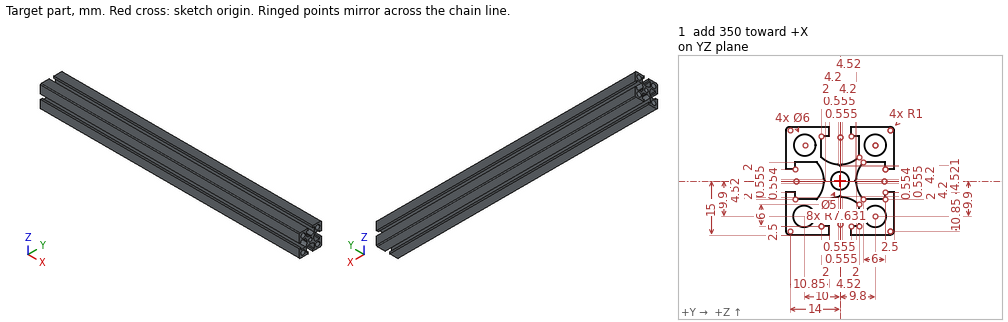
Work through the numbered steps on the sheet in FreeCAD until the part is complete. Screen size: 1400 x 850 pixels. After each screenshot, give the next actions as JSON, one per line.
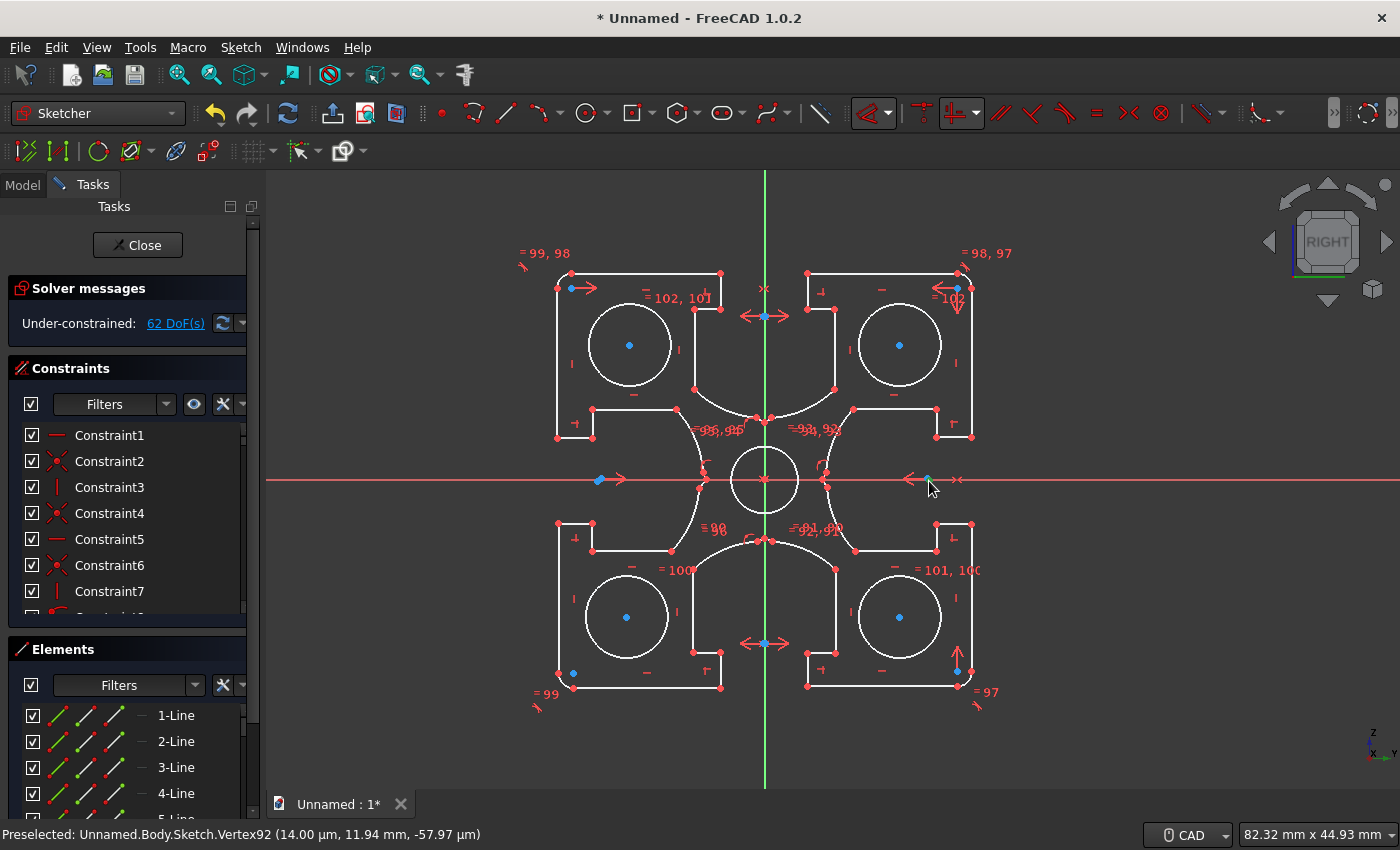
{"action": "scroll", "coordinate": [597, 481], "scroll_direction": "up", "scroll_amount": 6}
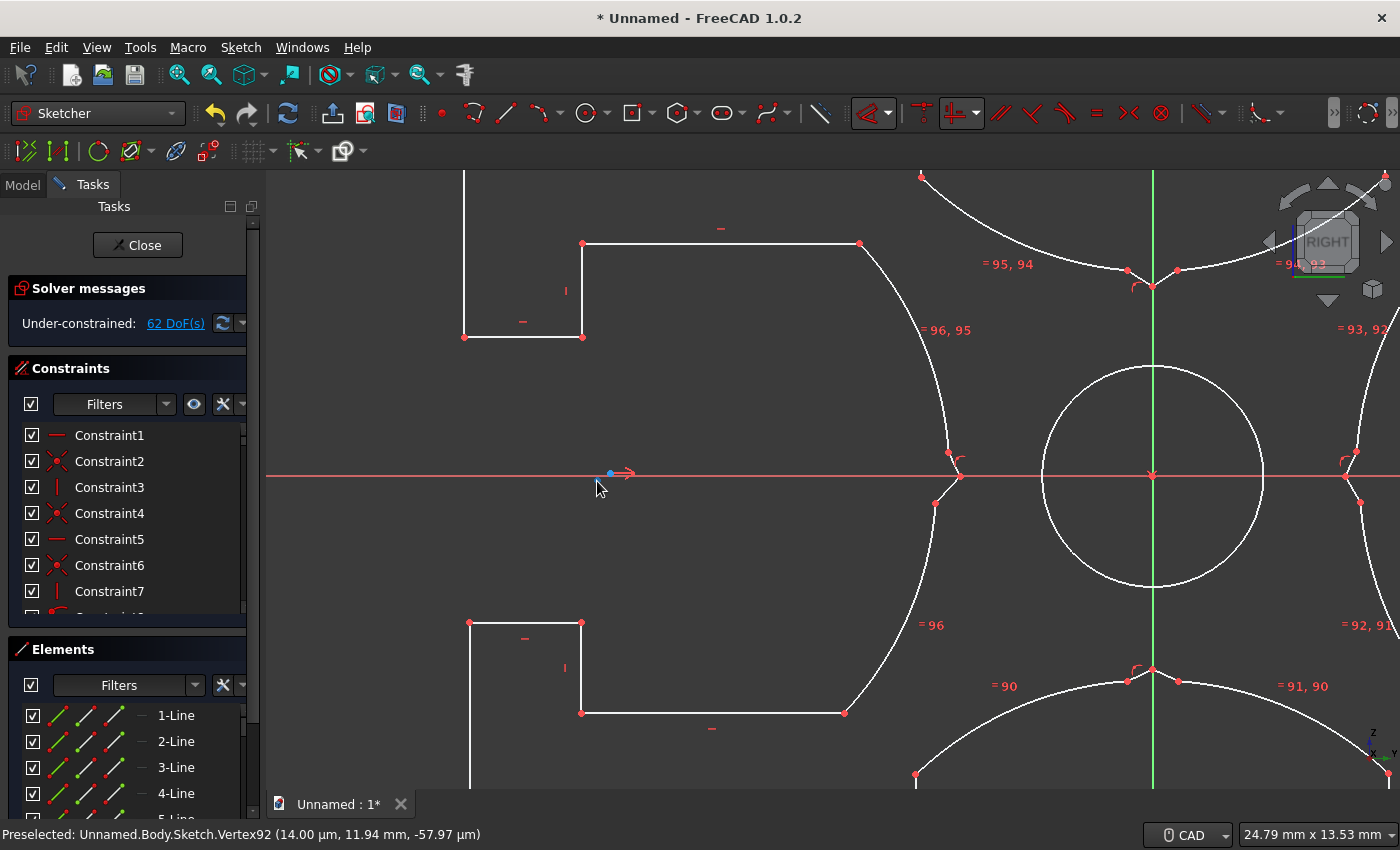
{"action": "left_click", "coordinate": [597, 481]}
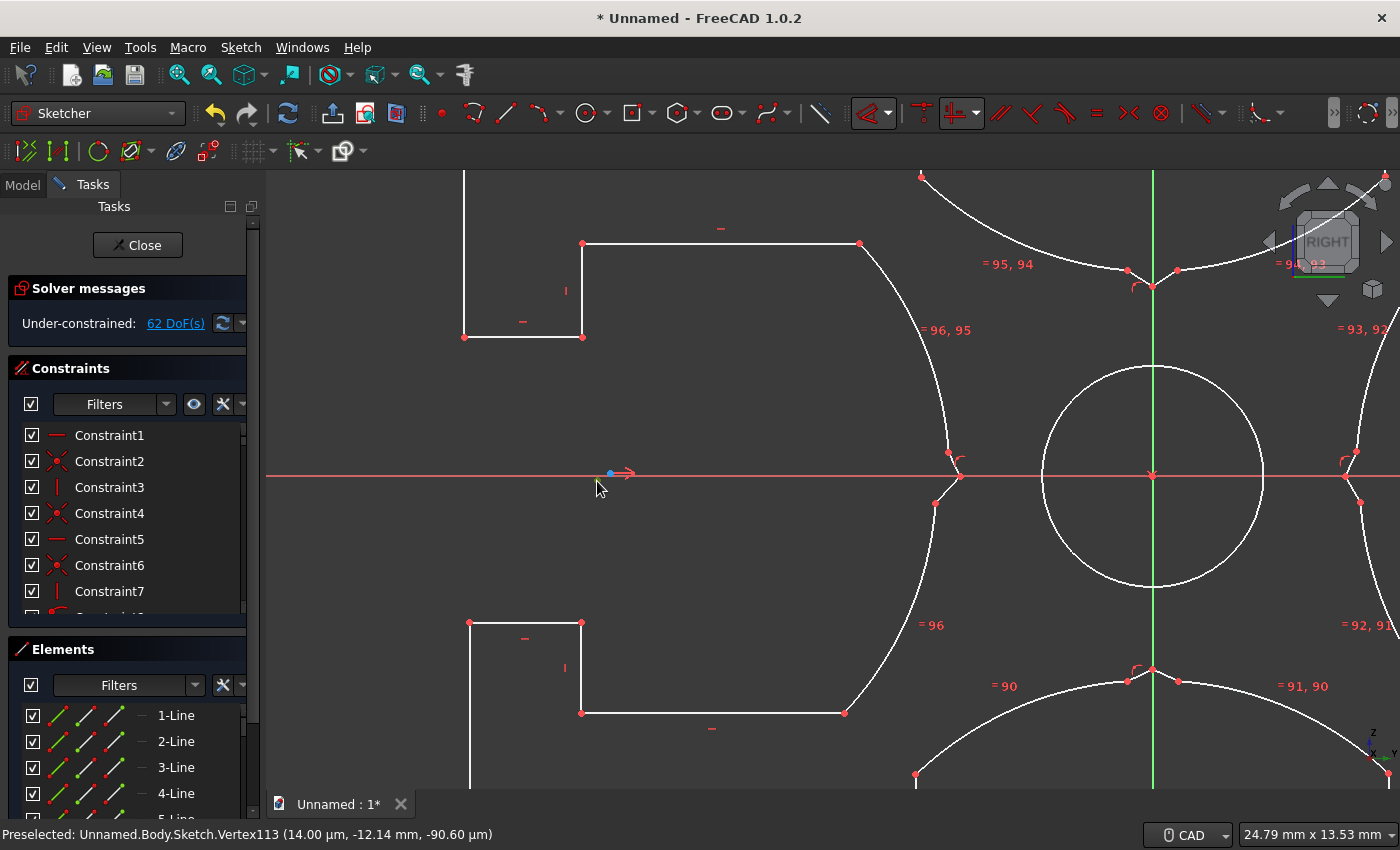
{"action": "left_click", "coordinate": [1153, 721]}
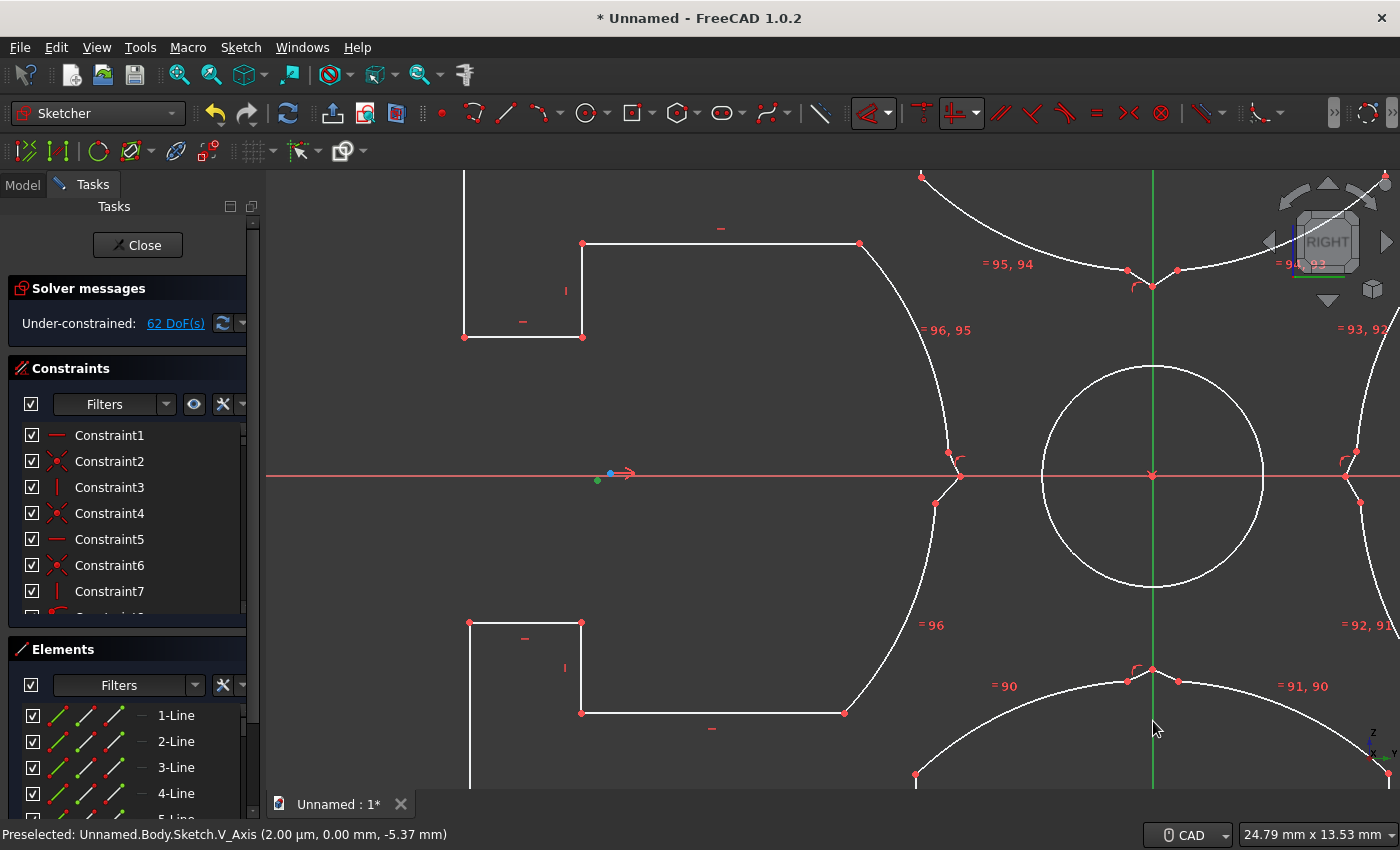
{"action": "left_click", "coordinate": [1130, 114]}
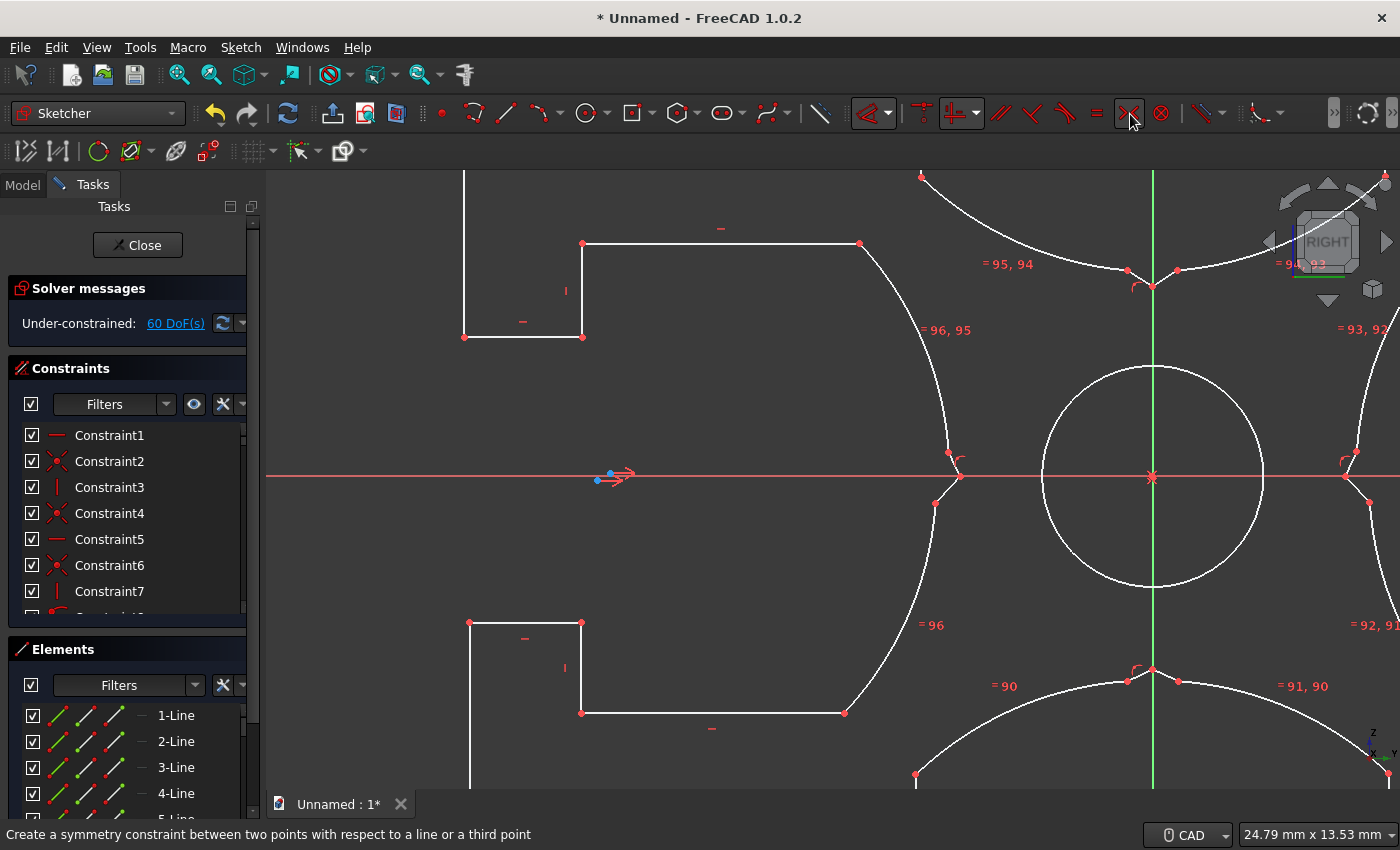
{"action": "scroll", "coordinate": [597, 481], "scroll_direction": "down", "scroll_amount": 6}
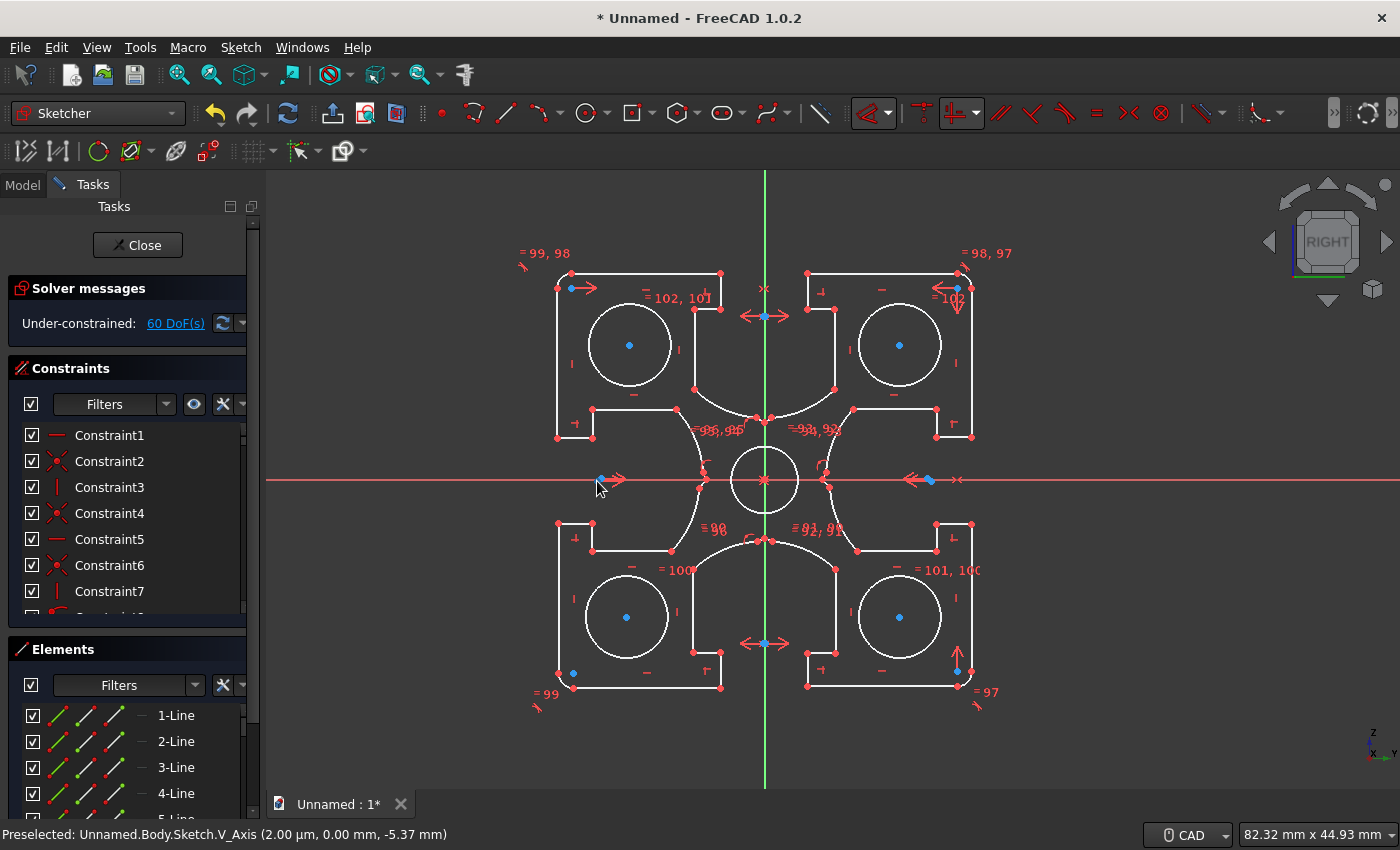
{"action": "left_click", "coordinate": [957, 672]}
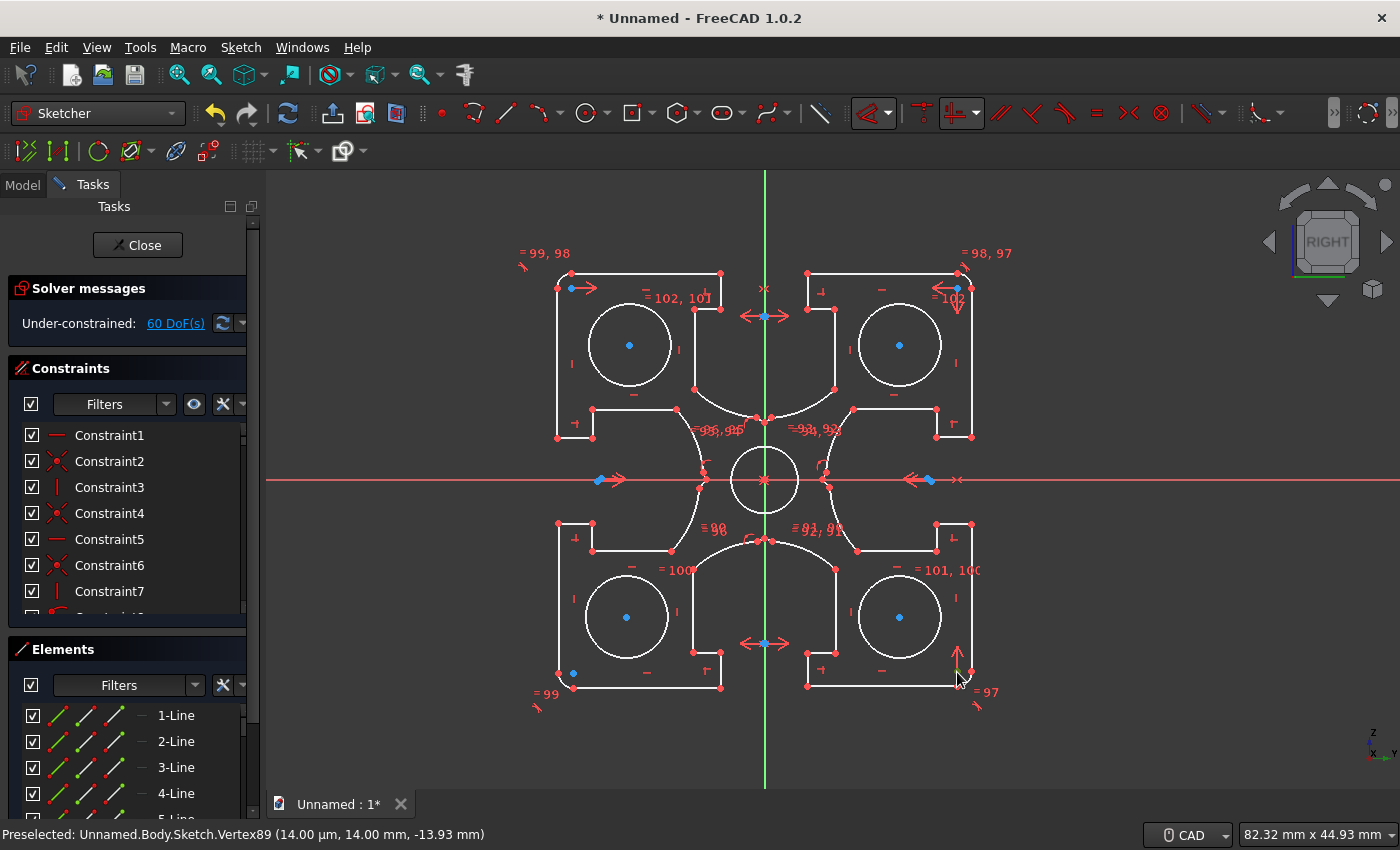
{"action": "left_click", "coordinate": [573, 674]}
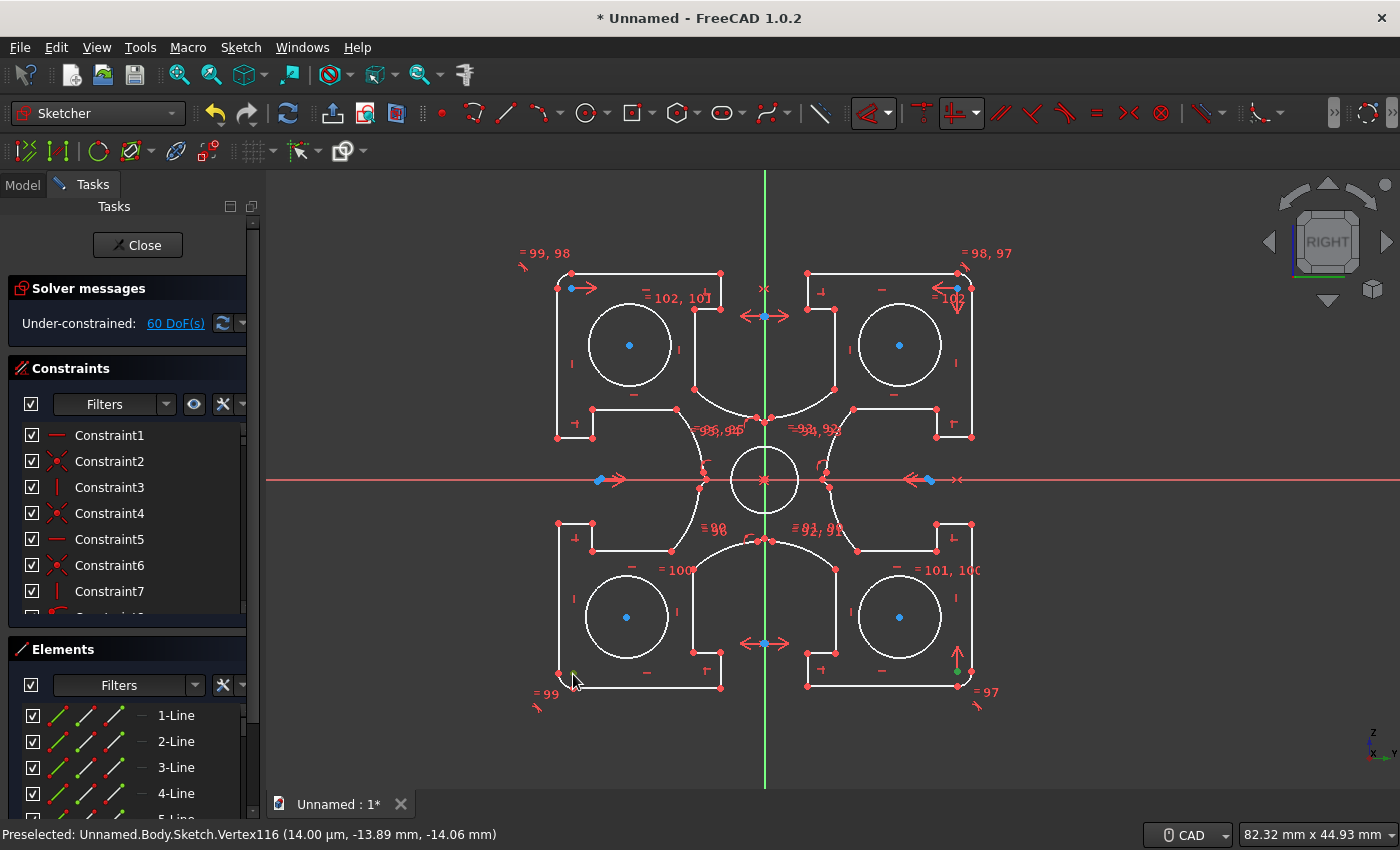
{"action": "left_click", "coordinate": [765, 721]}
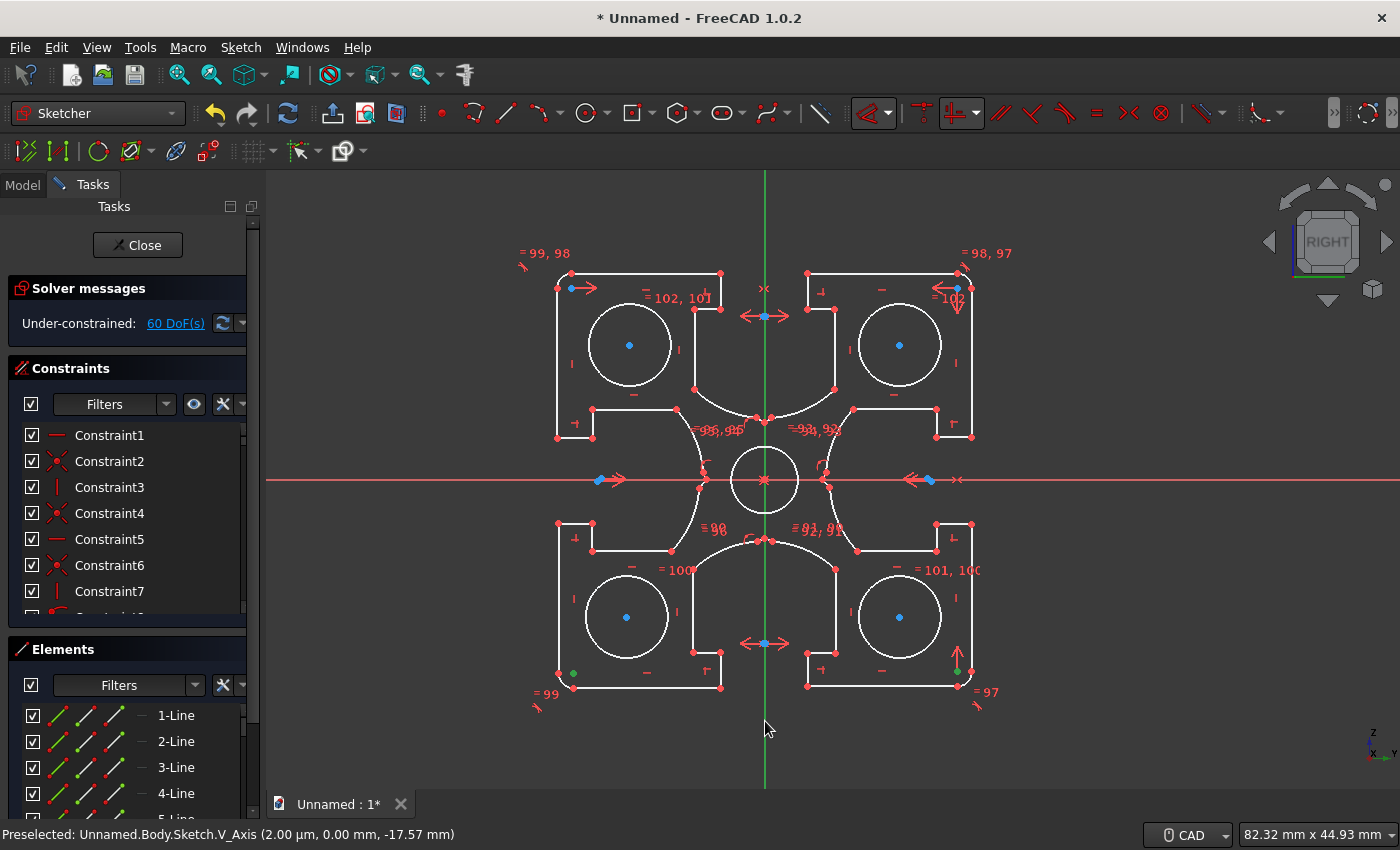
{"action": "key", "text": "s"}